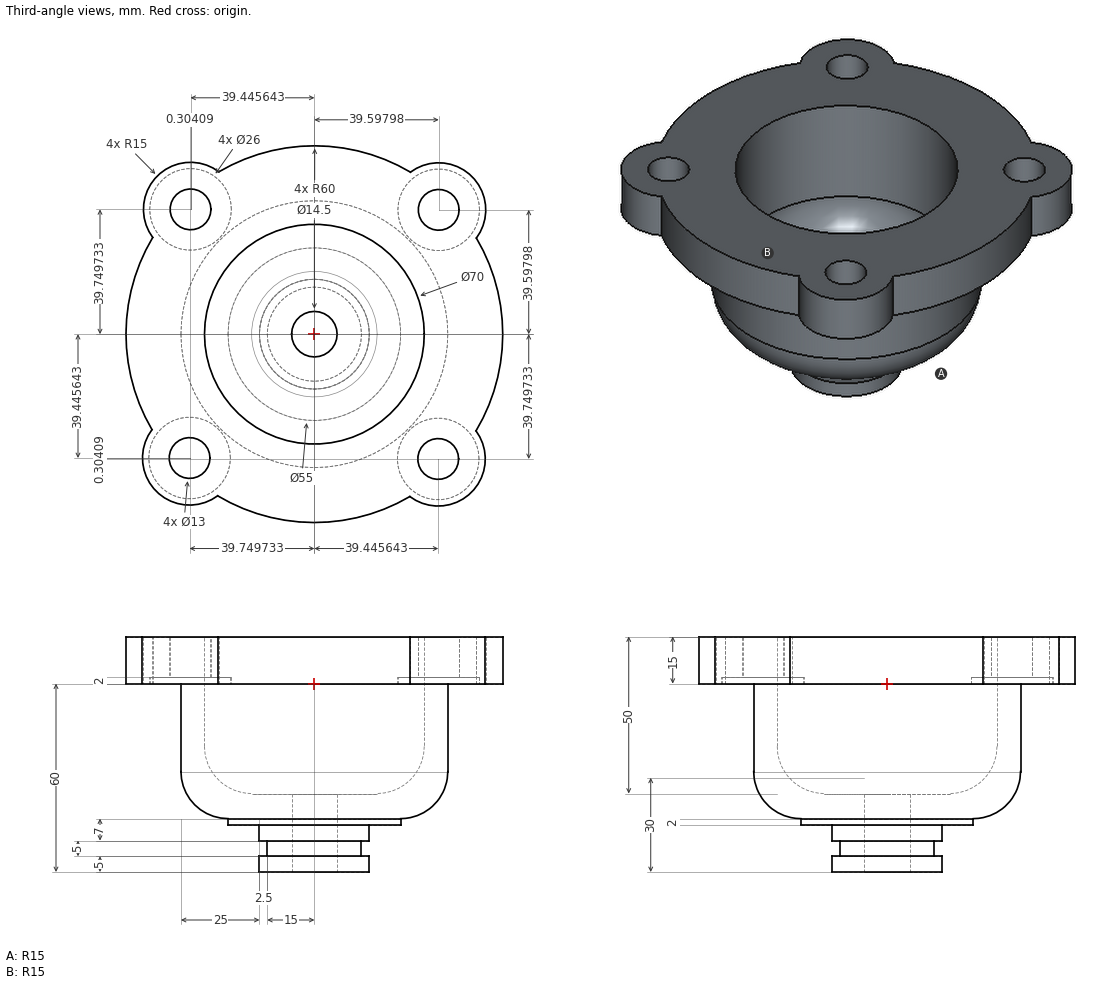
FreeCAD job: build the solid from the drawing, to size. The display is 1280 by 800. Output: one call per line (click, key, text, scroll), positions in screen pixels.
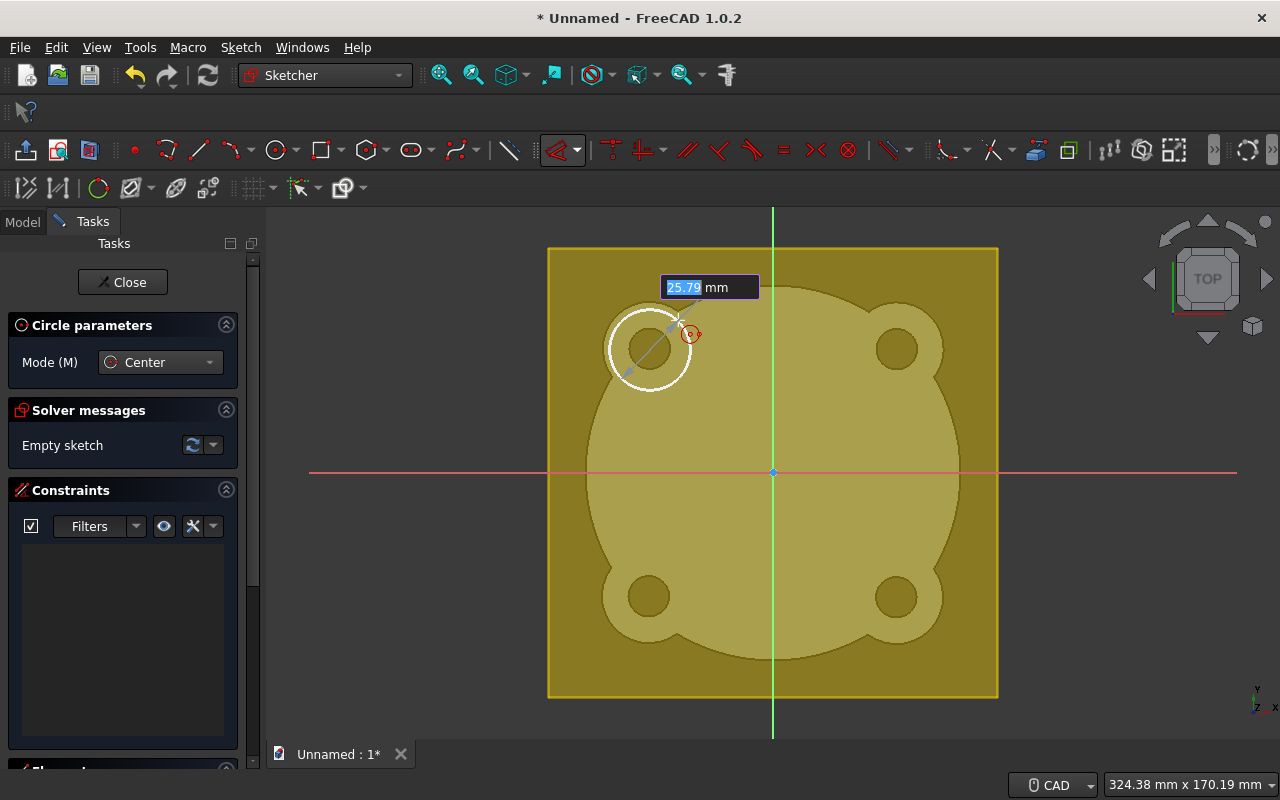
text(26)
key(Return)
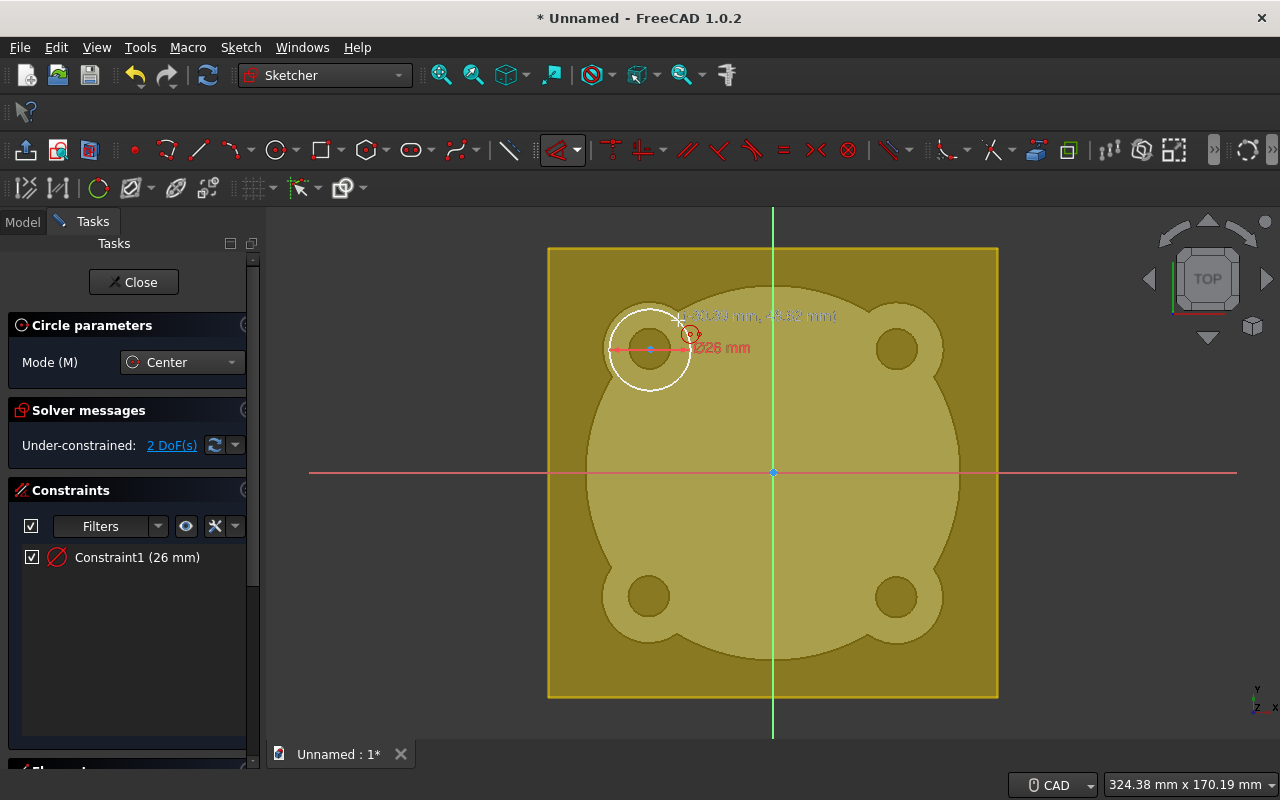
click(897, 349)
move(926, 320)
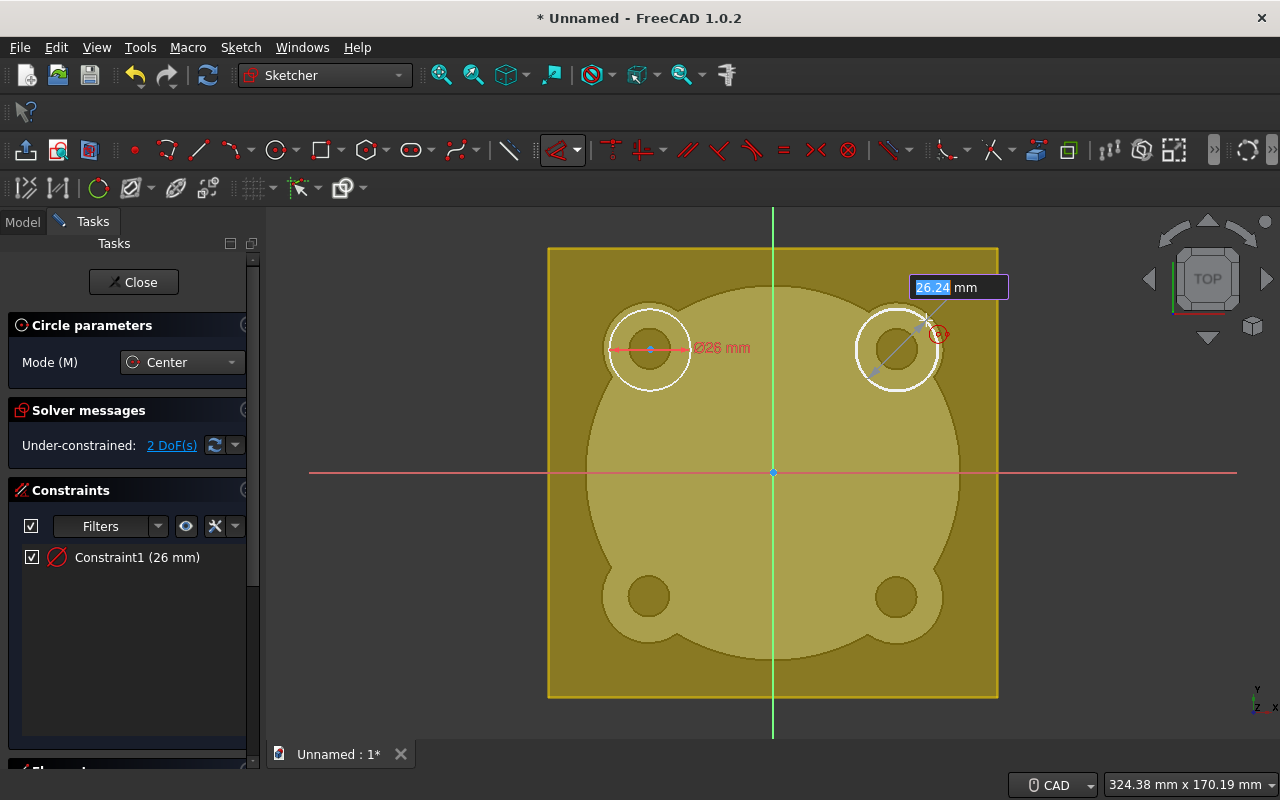
text(26)
key(Return)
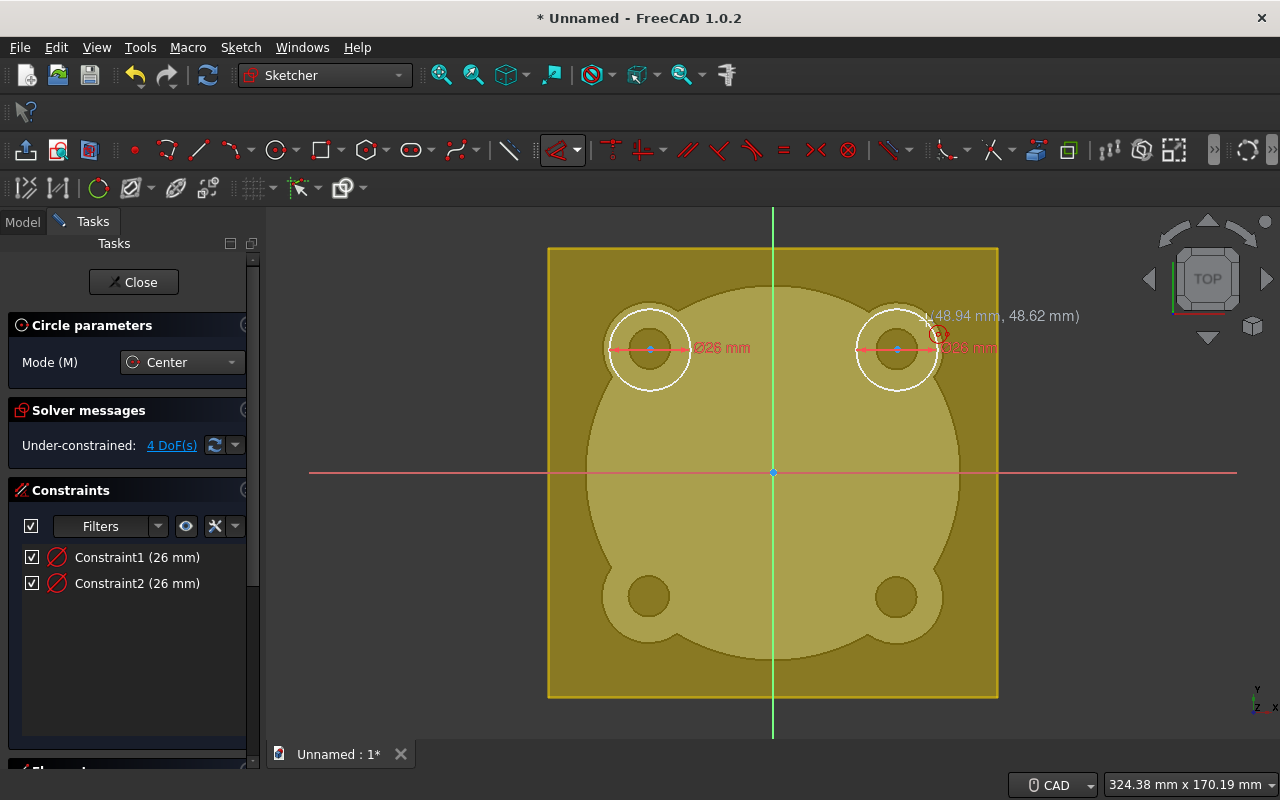
click(896, 597)
move(925, 569)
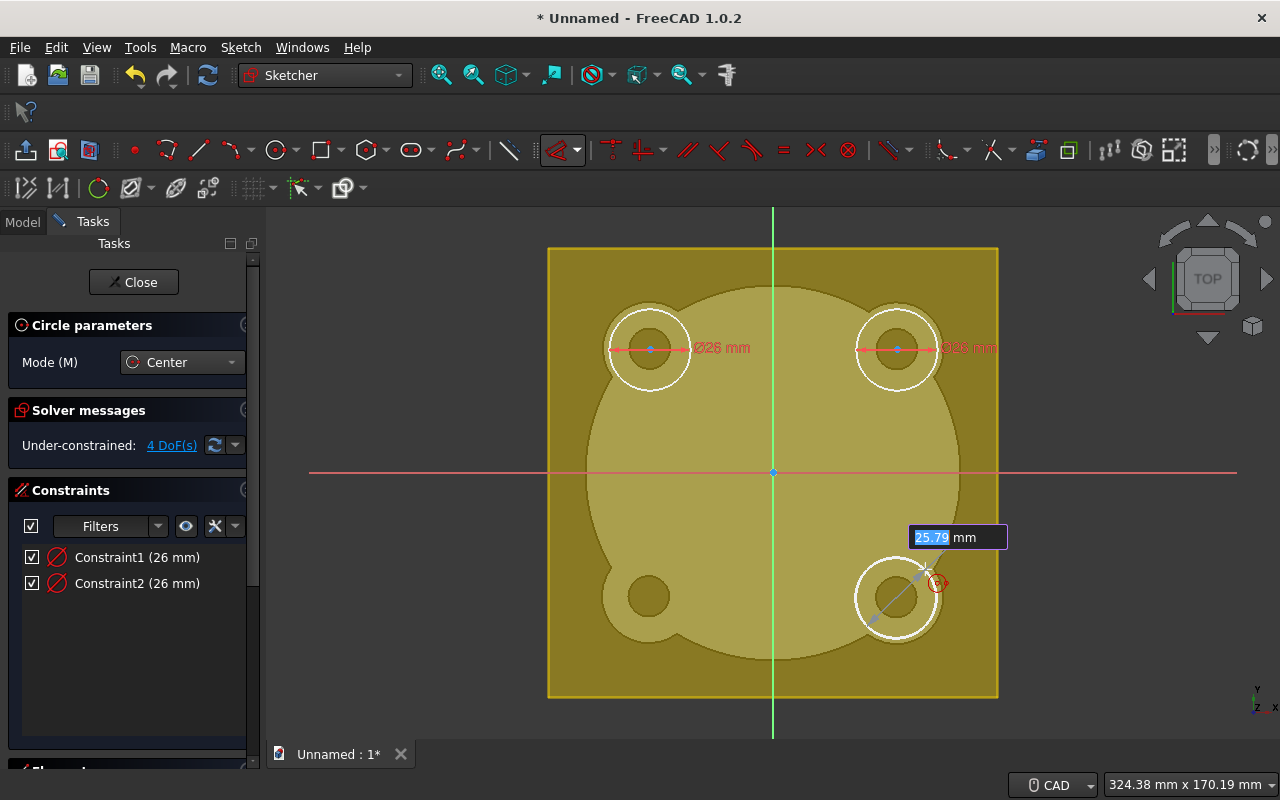
text(26)
key(Return)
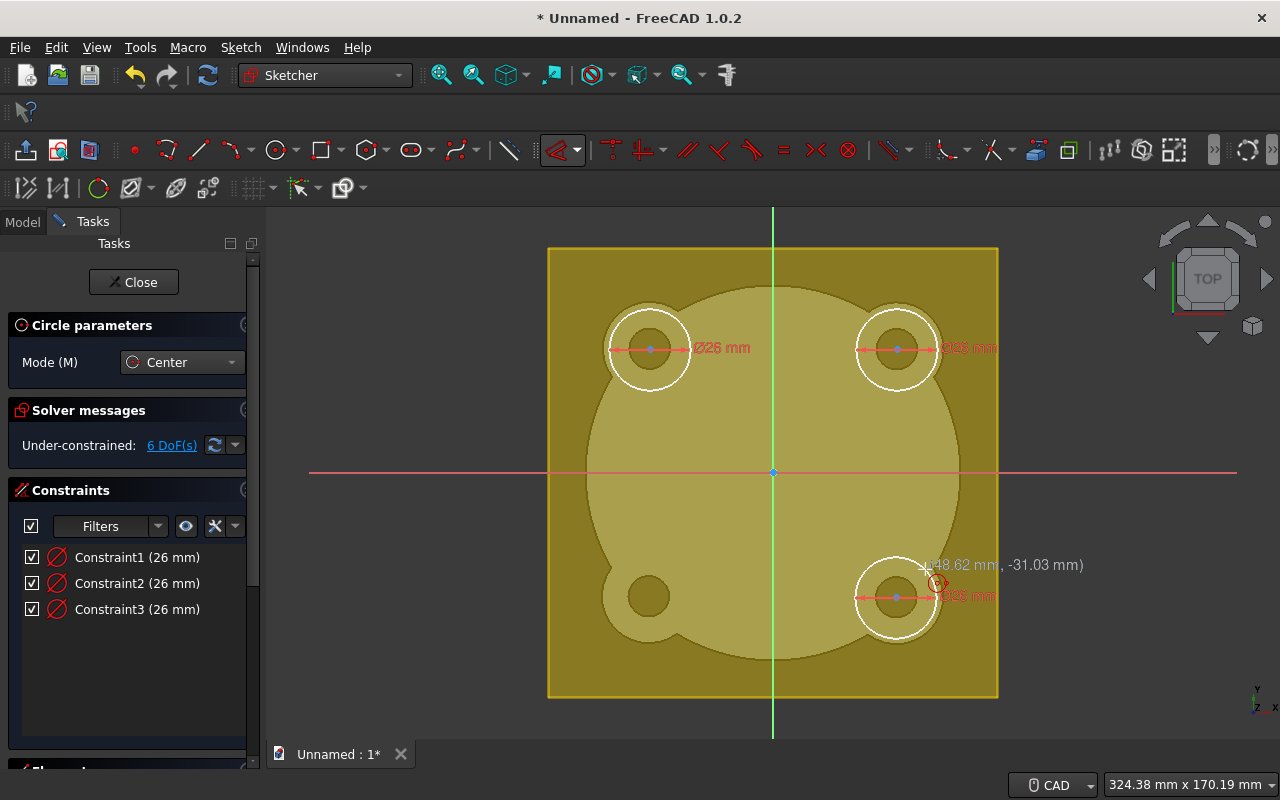
click(649, 596)
move(677, 568)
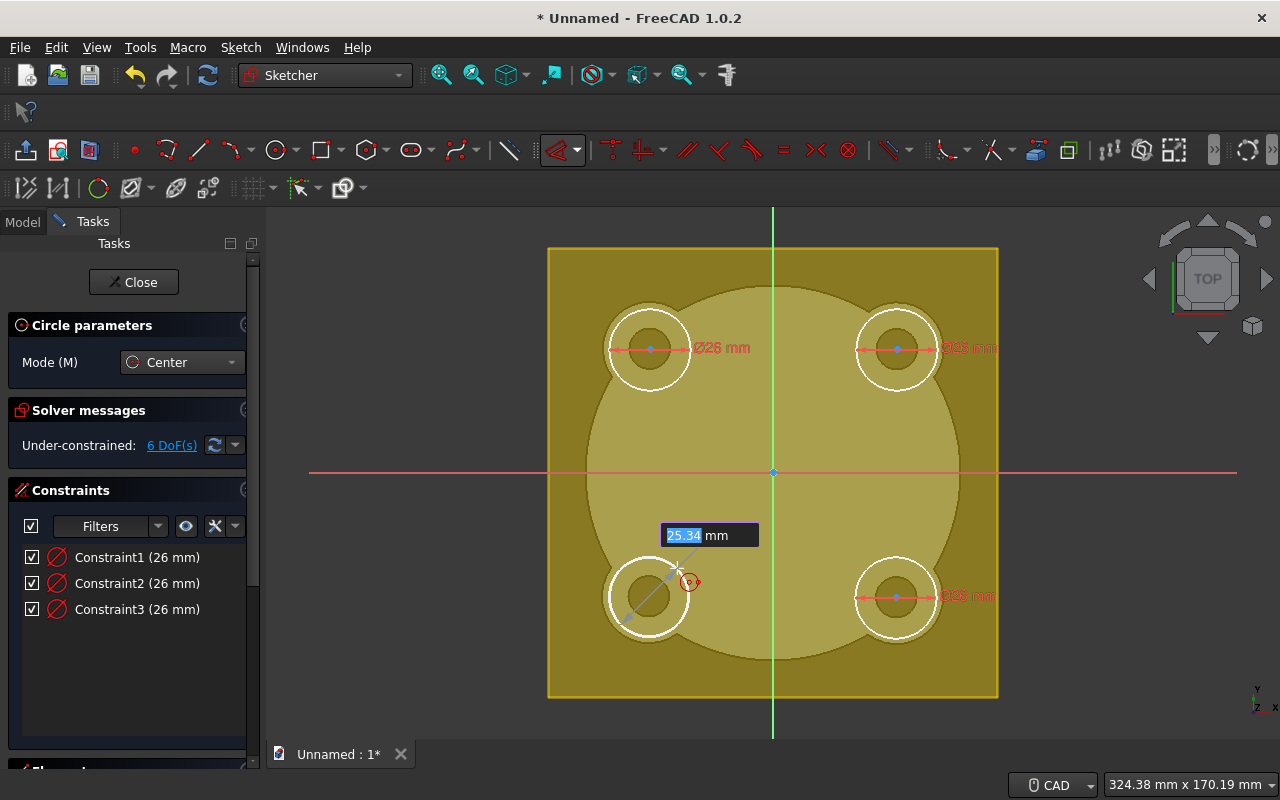
text(26)
key(Return)
key(Escape)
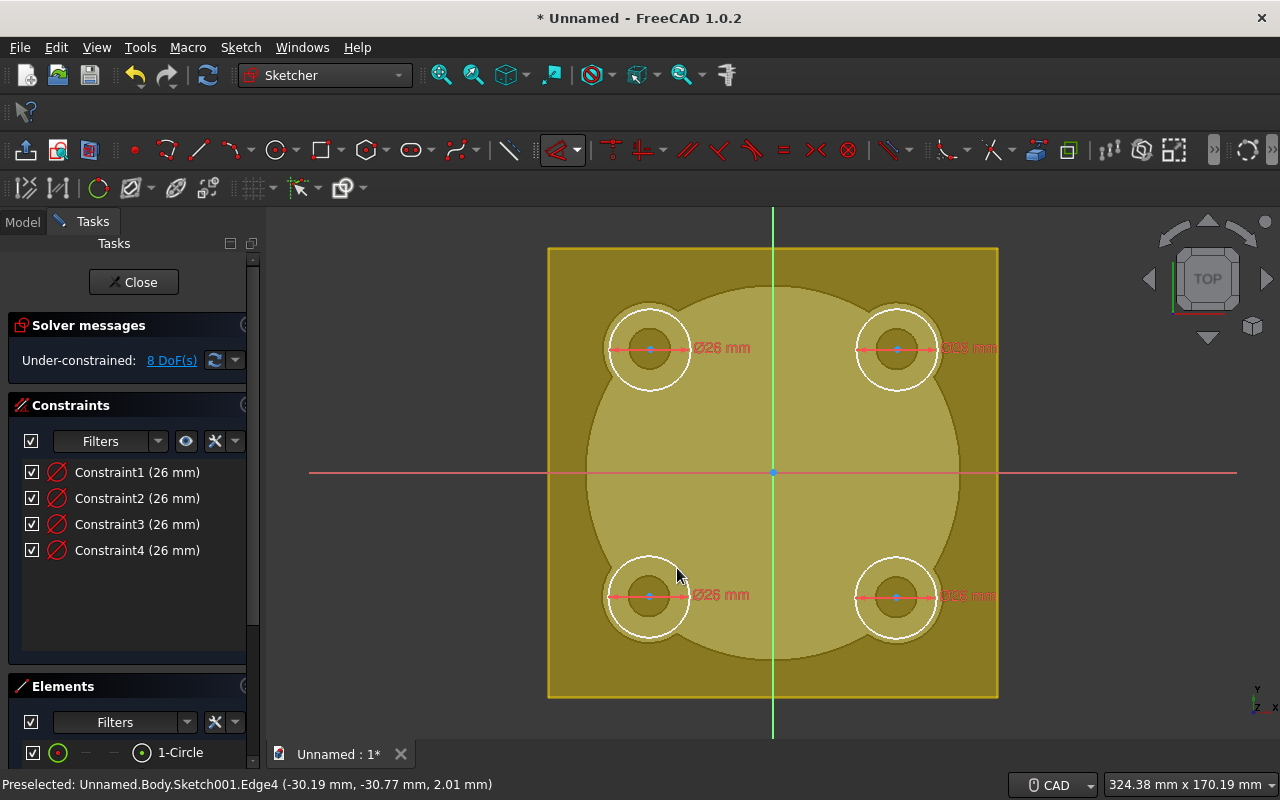
click(897, 350)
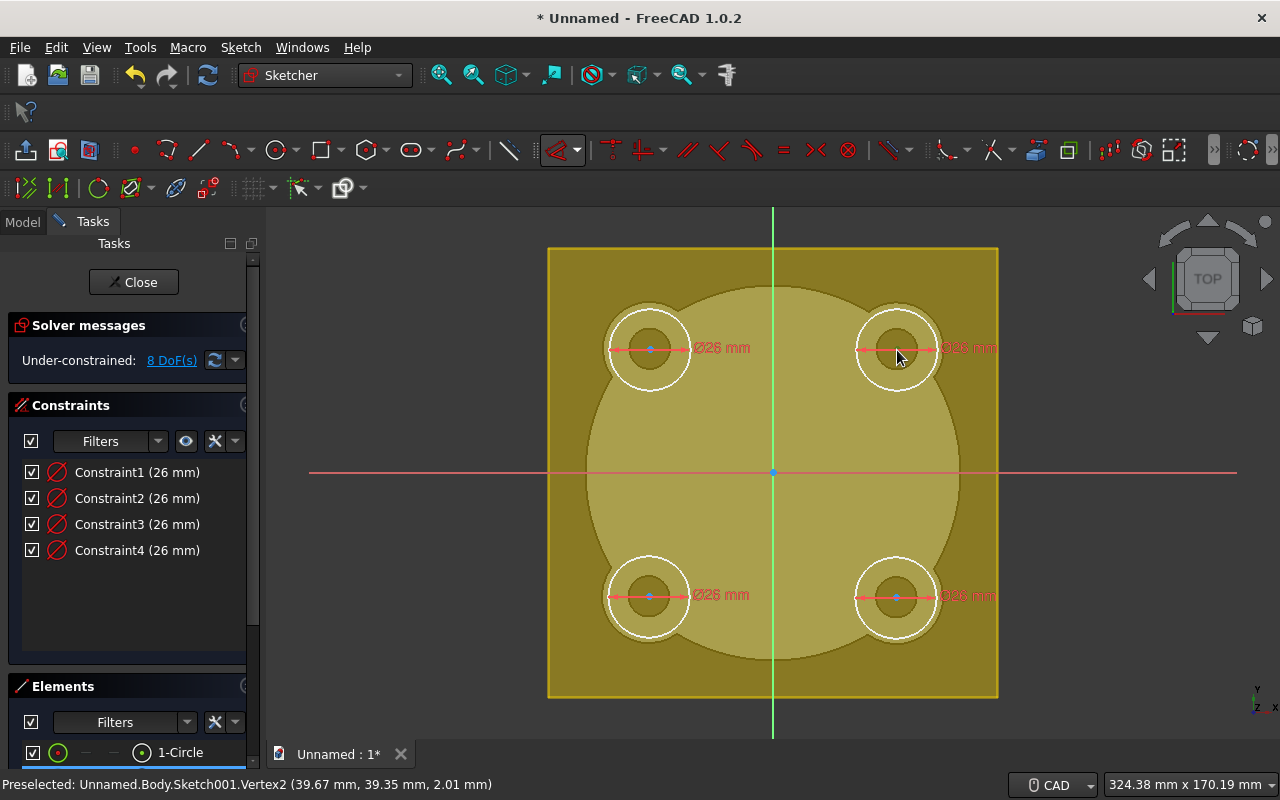
key(l)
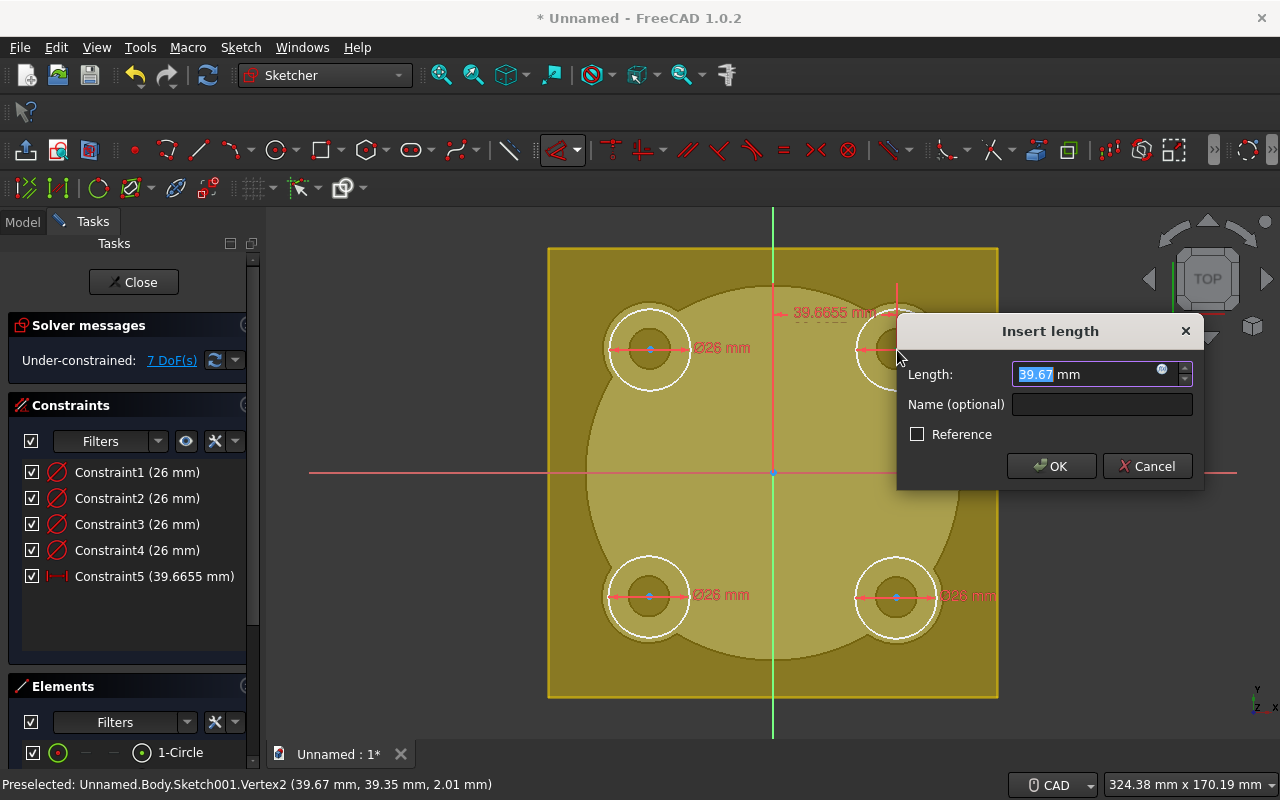
text(39.59798)
key(Return)